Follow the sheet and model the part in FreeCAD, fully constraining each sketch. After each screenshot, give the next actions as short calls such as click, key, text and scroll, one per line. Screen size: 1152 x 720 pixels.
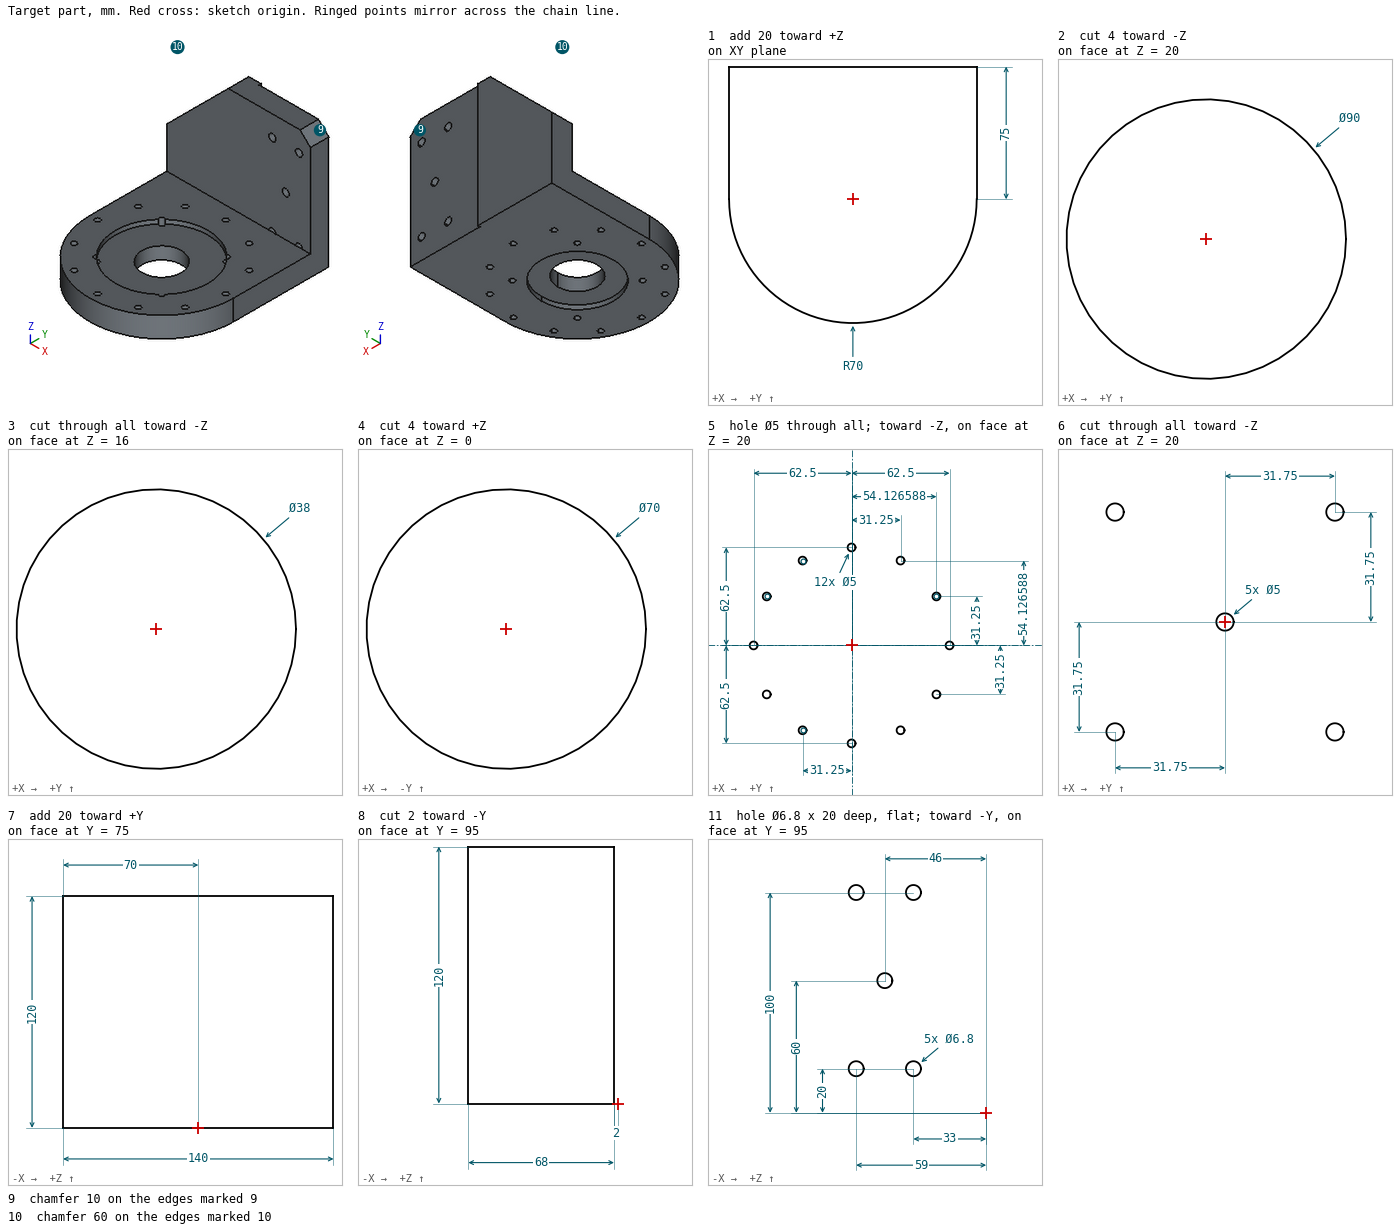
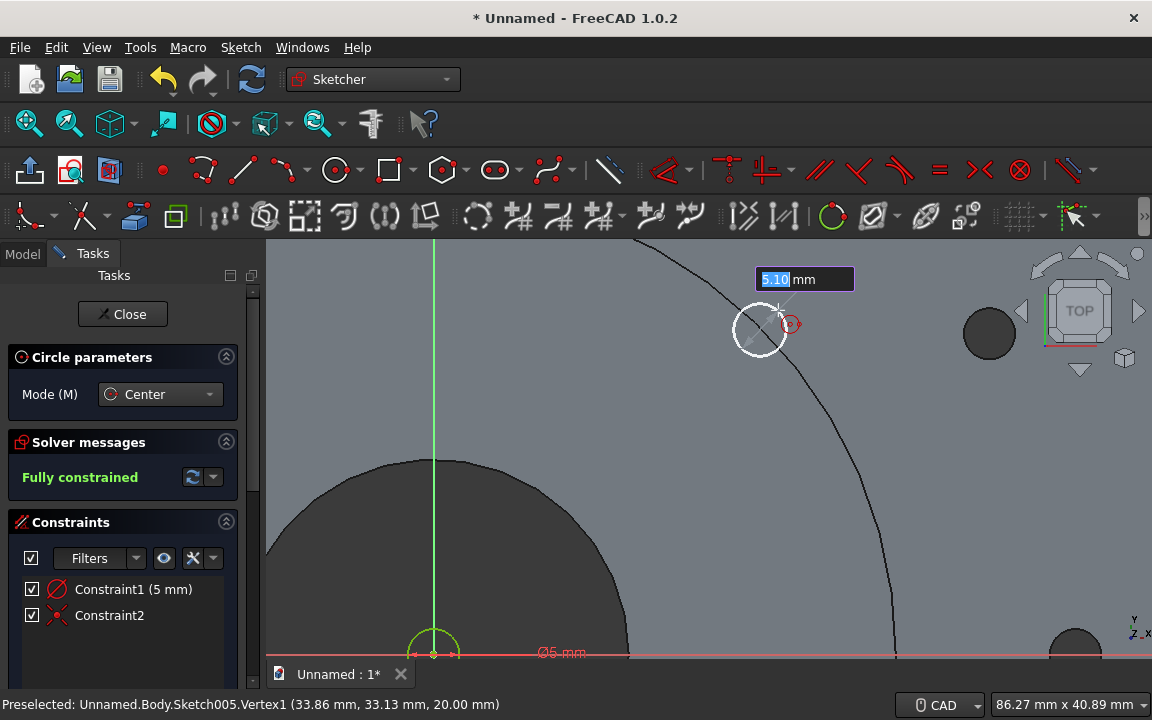
text(5)
key(Return)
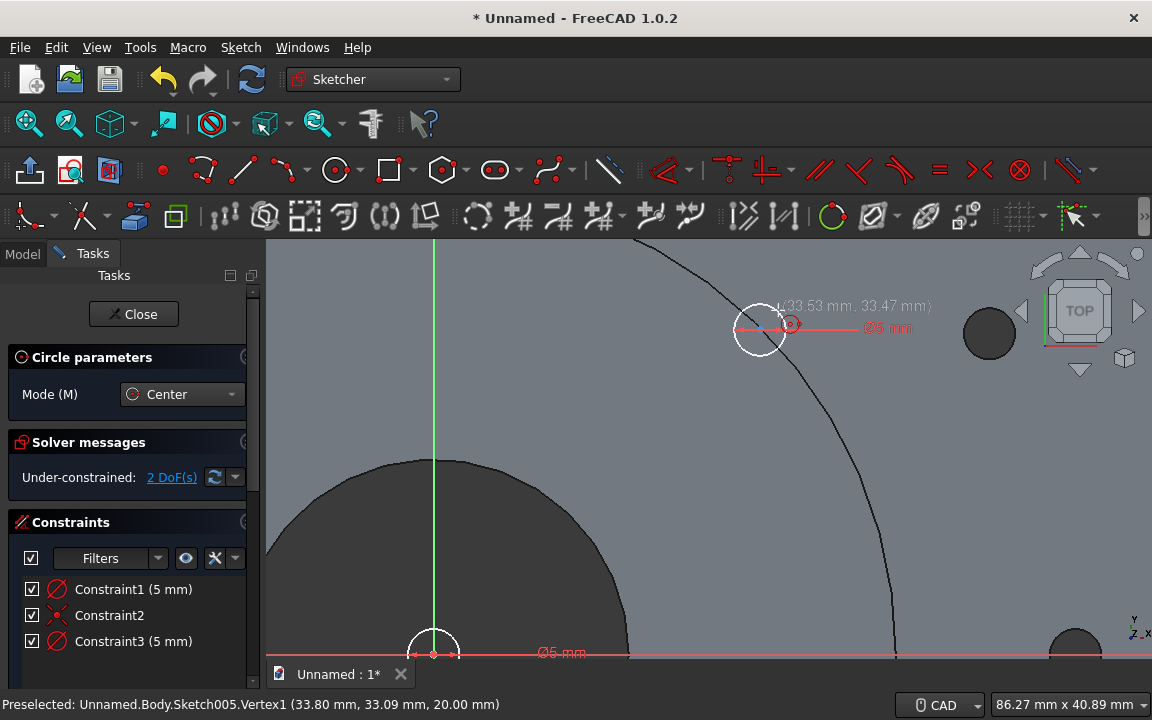
scroll(761, 329, down, 5)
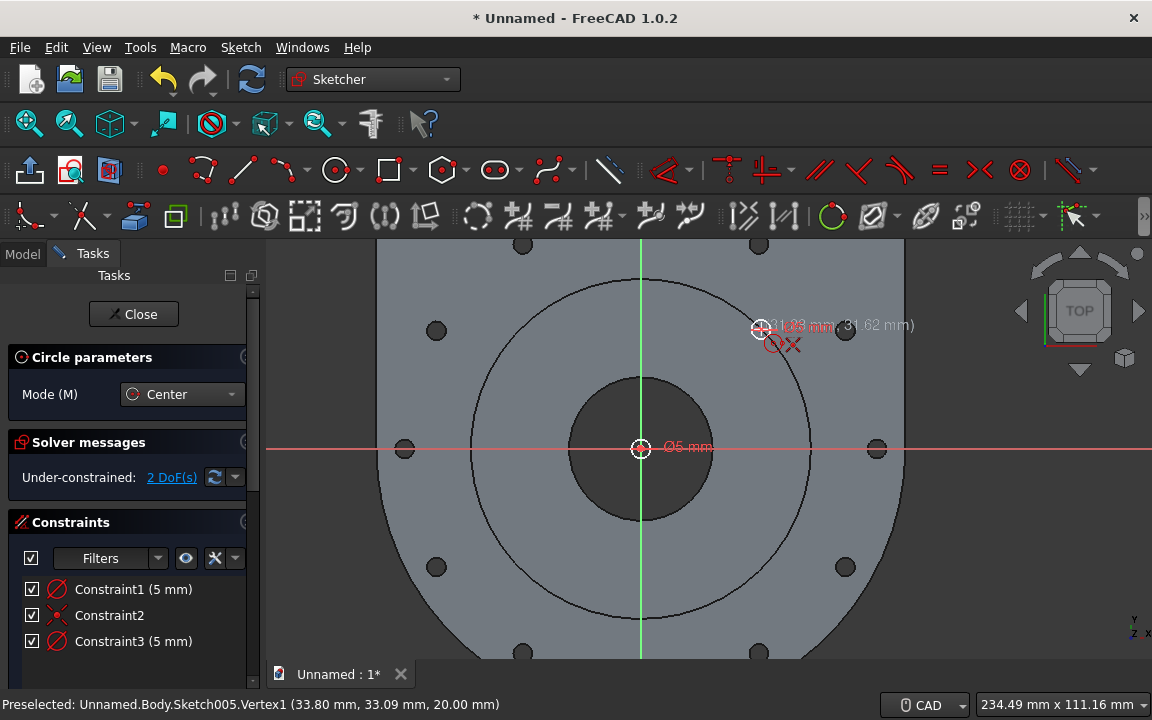
scroll(521, 569, up, 5)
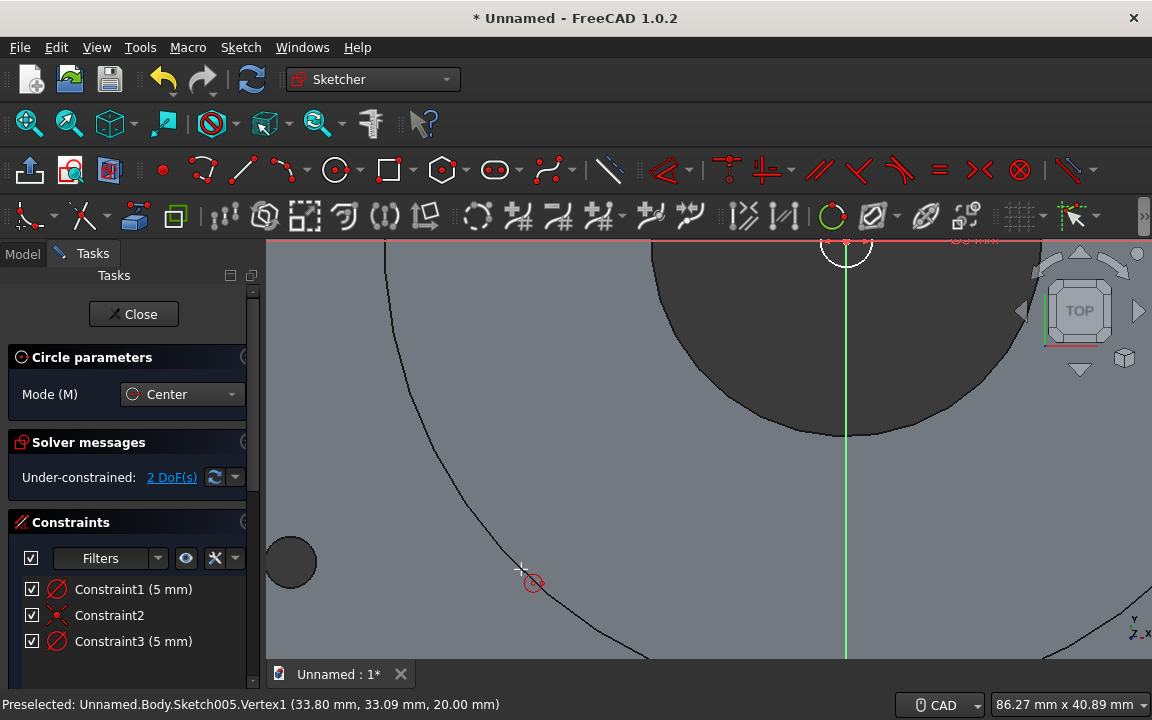
click(520, 567)
move(539, 549)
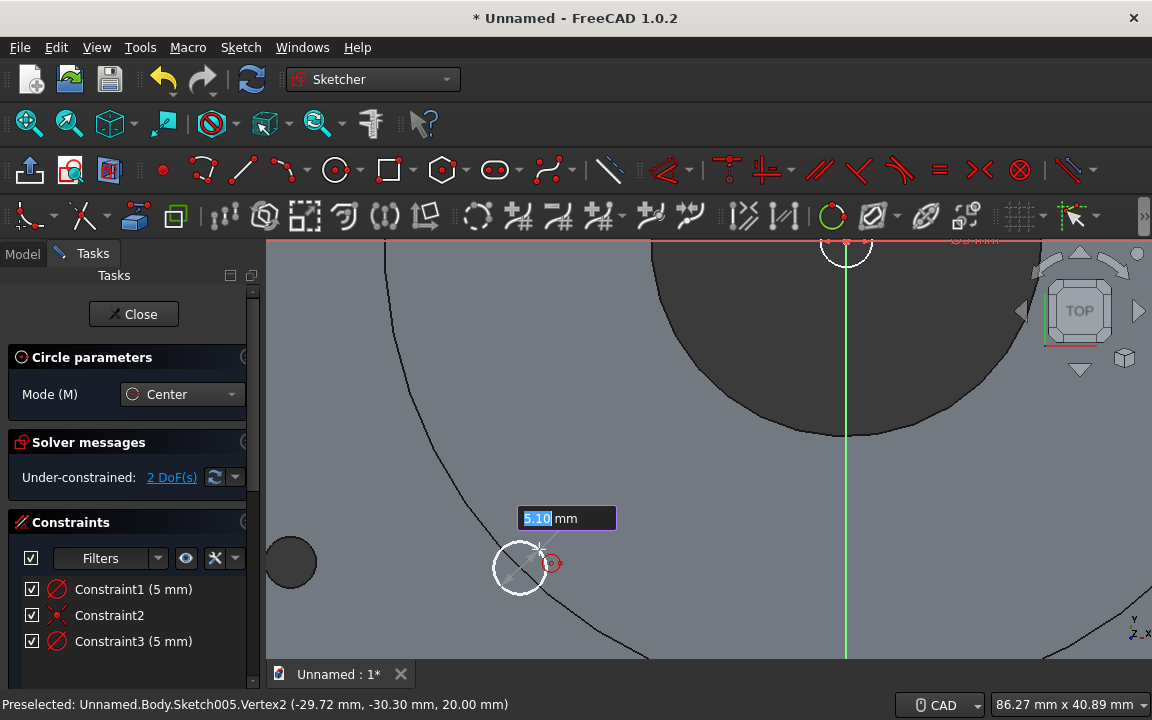
text(5)
key(Return)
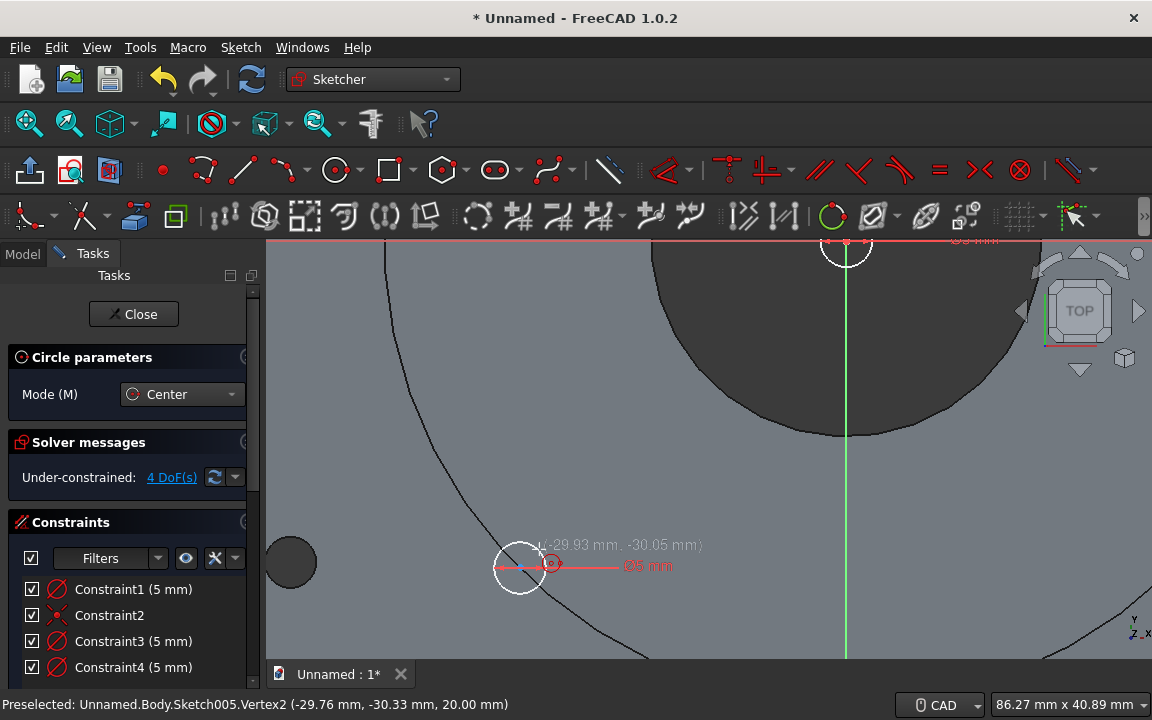
scroll(521, 570, down, 5)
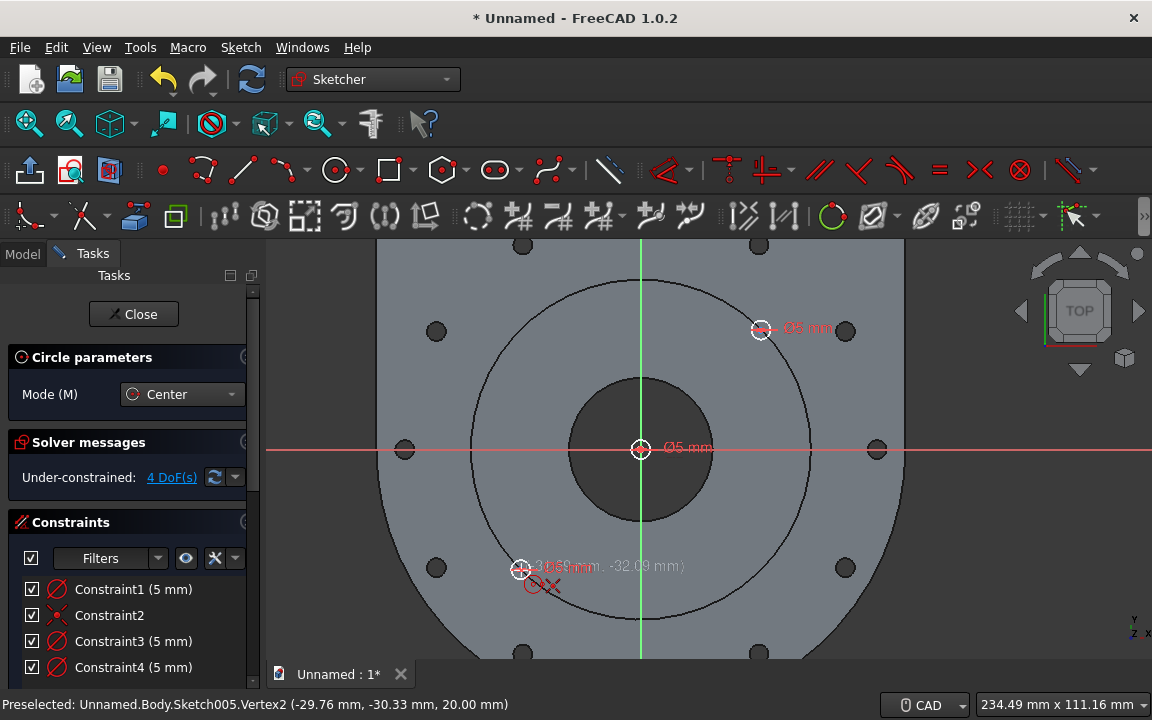
scroll(521, 330, up, 5)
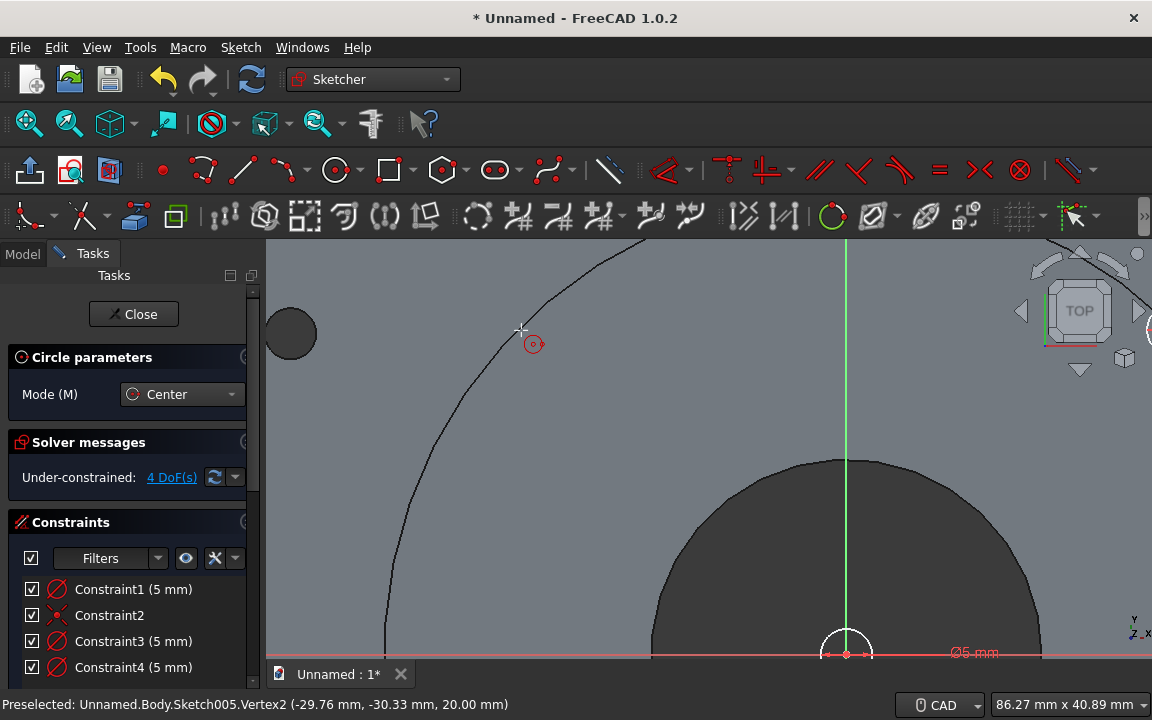
click(520, 329)
move(539, 310)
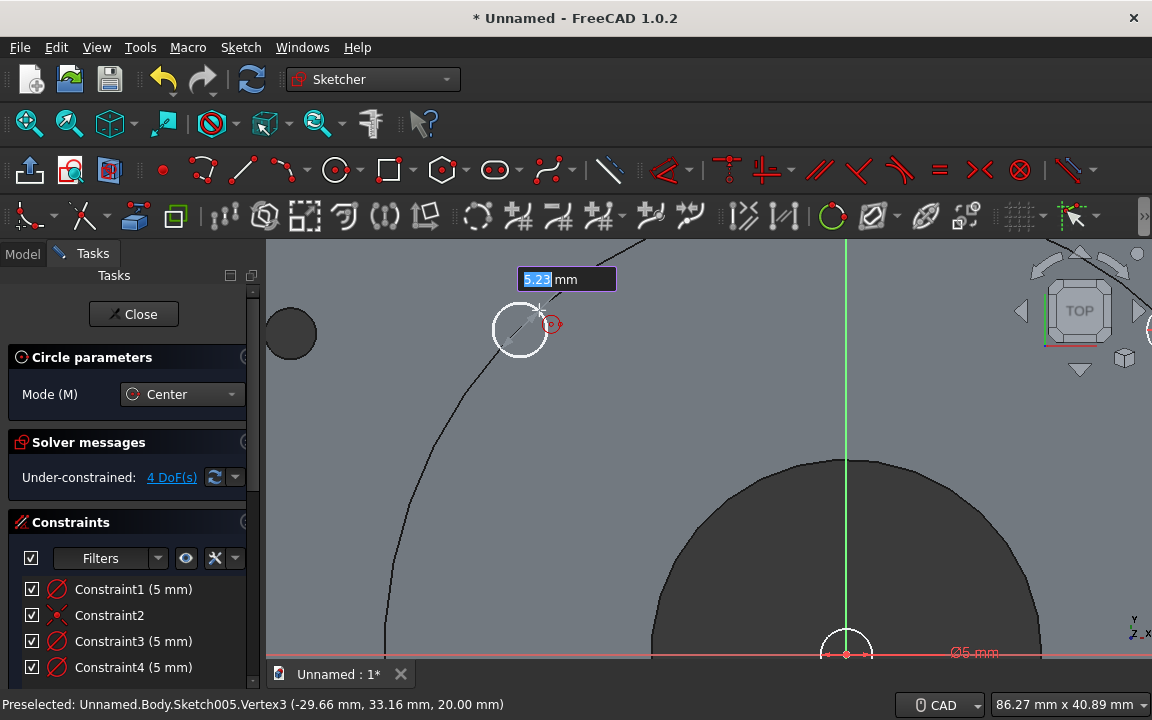
text(5)
key(Return)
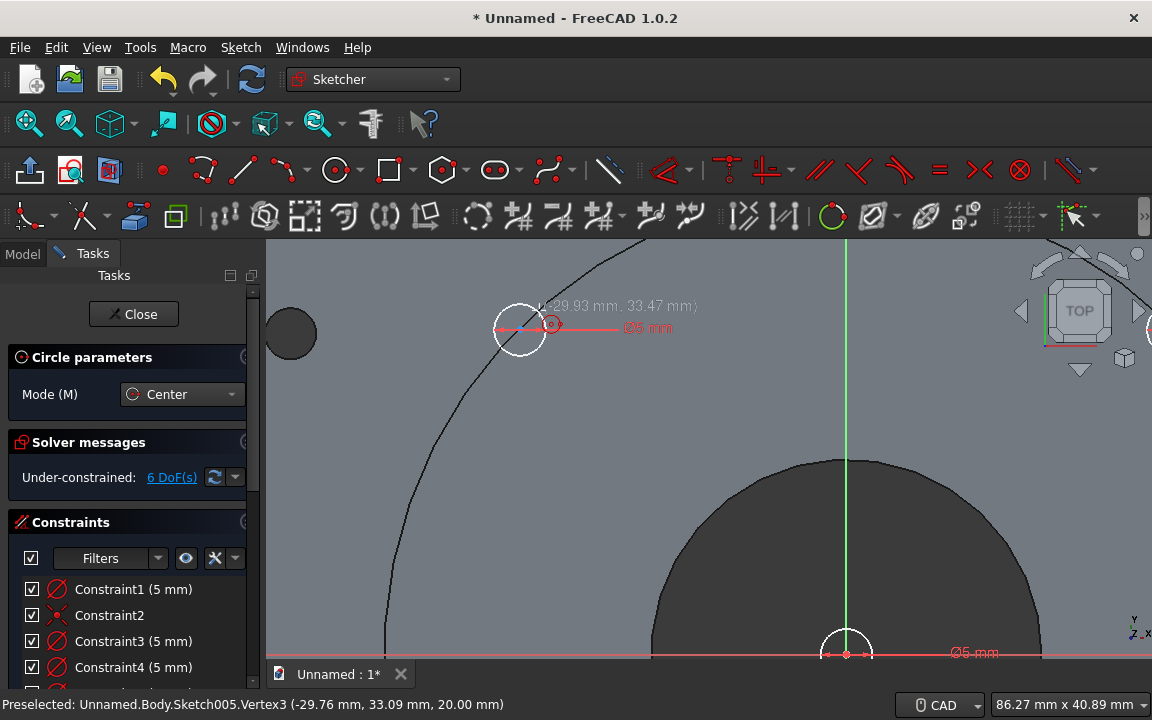
scroll(521, 329, down, 5)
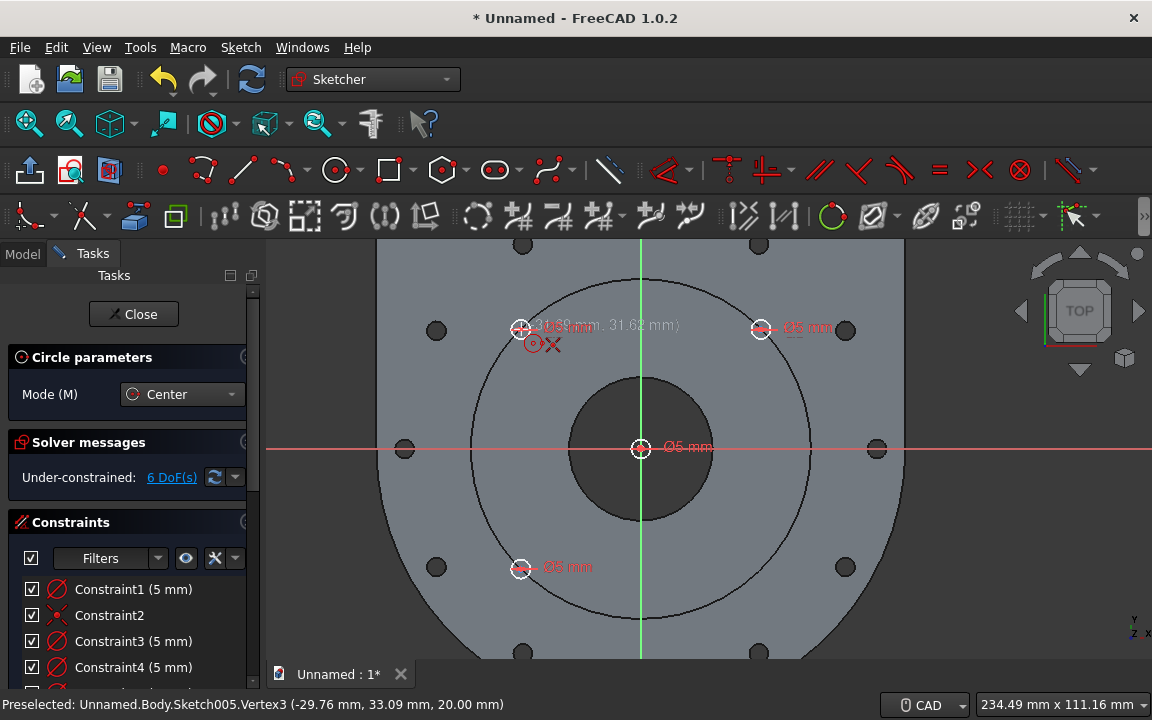
scroll(761, 569, up, 5)